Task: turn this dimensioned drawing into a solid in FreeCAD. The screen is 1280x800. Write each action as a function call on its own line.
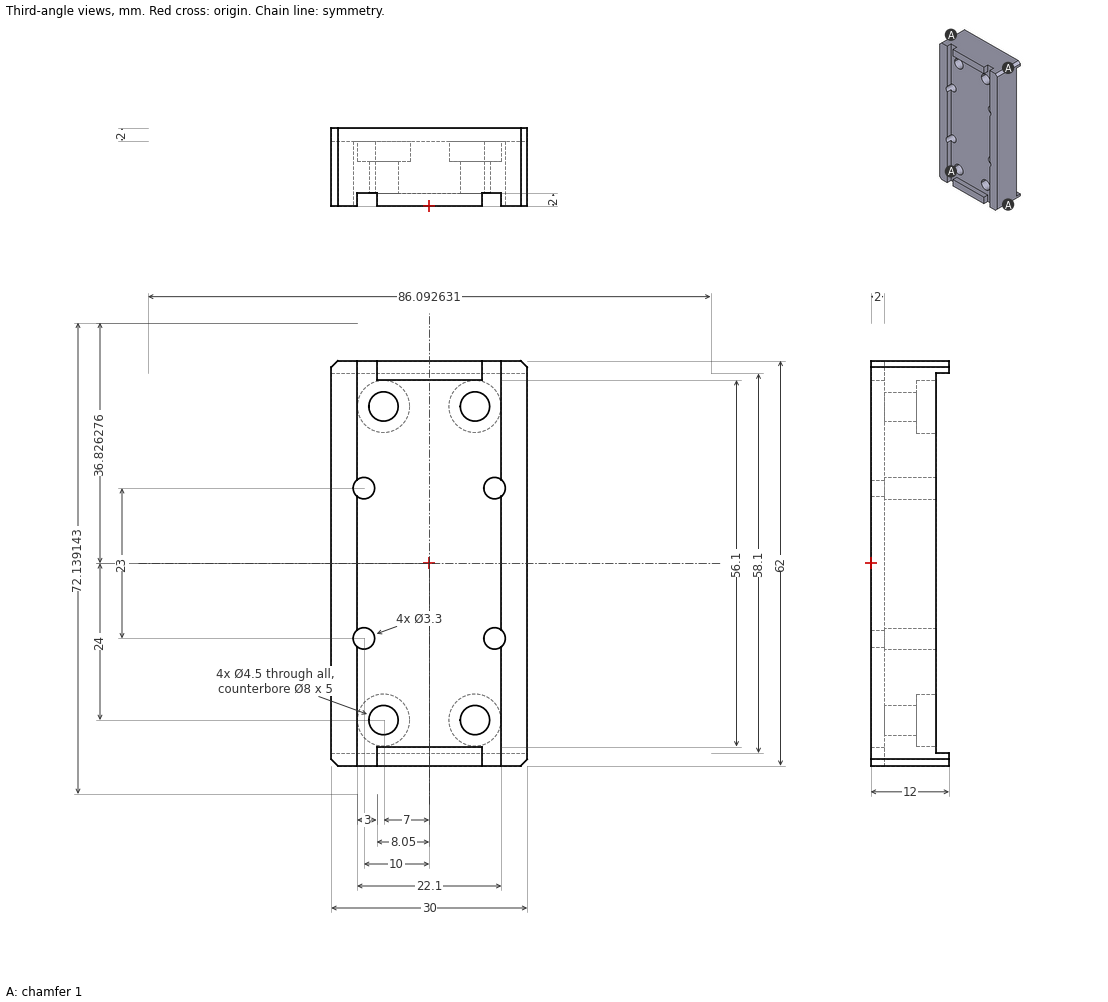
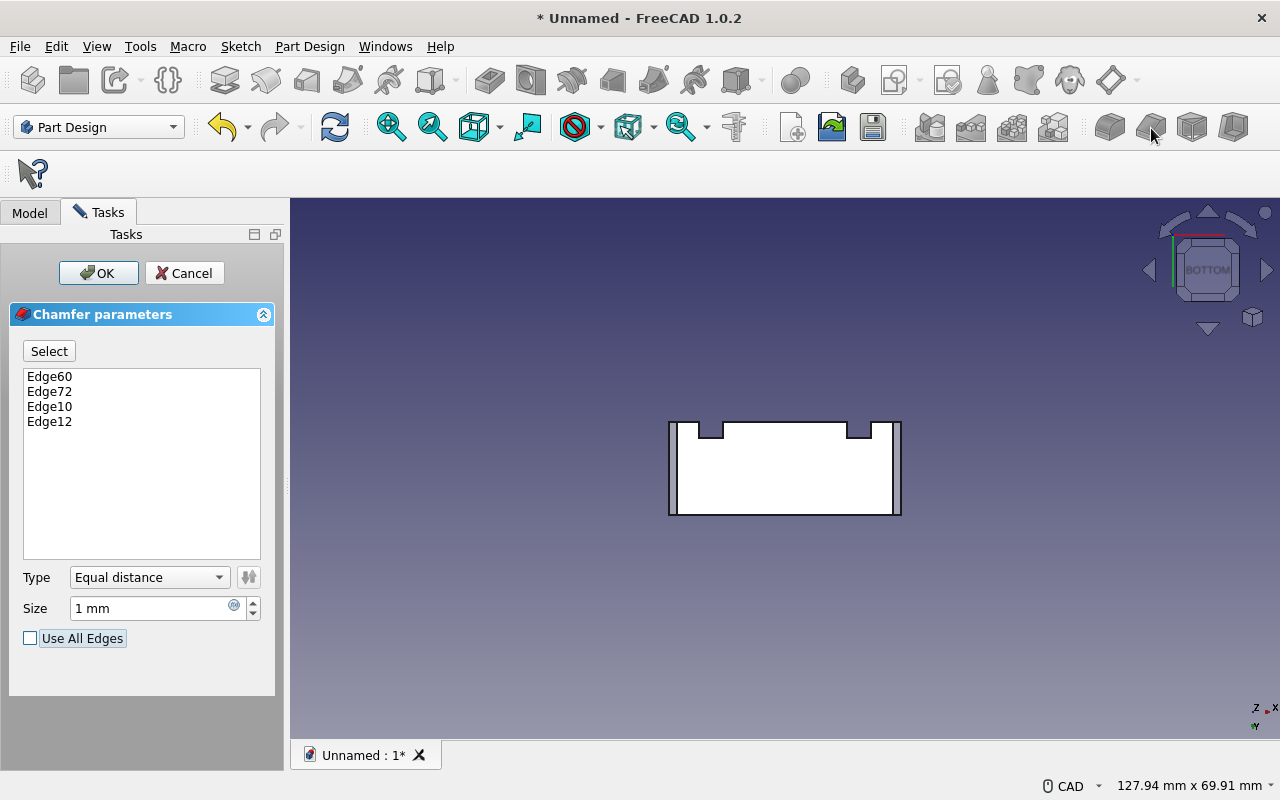
click(99, 273)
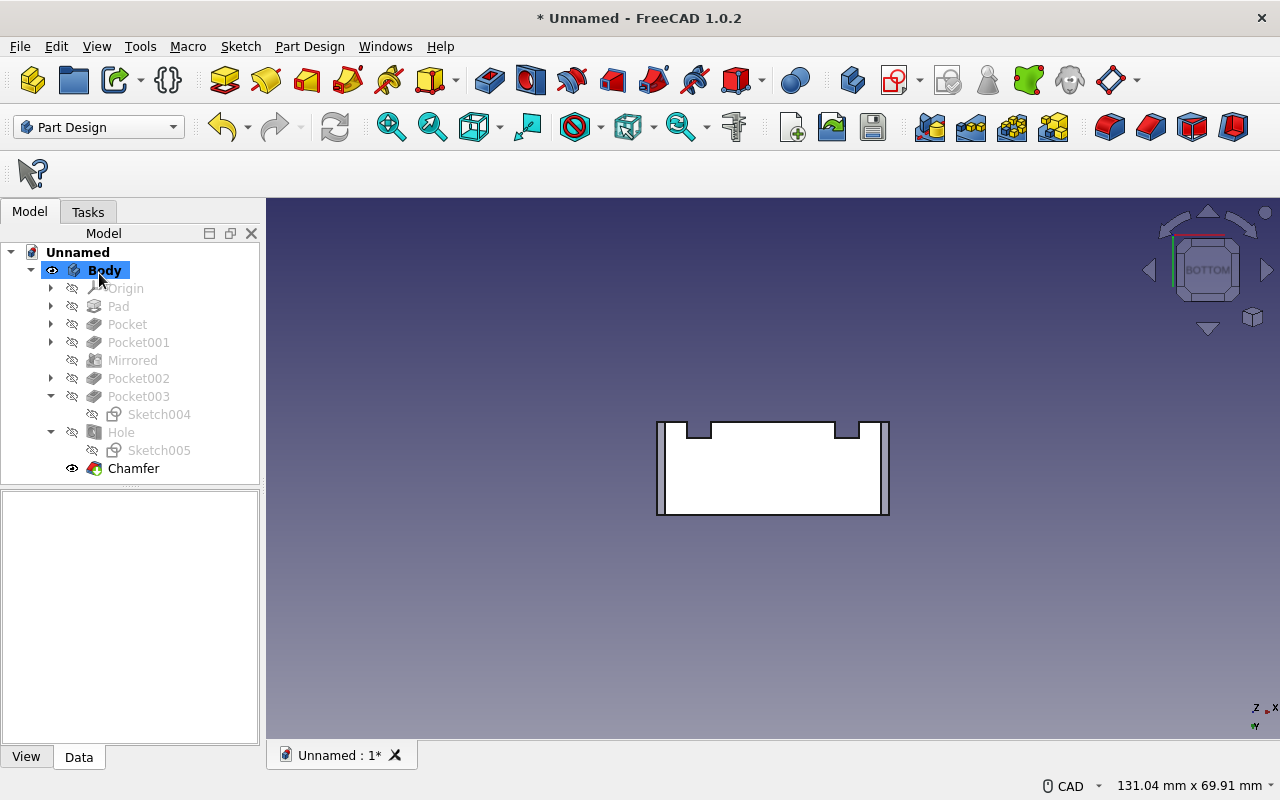
key(0)